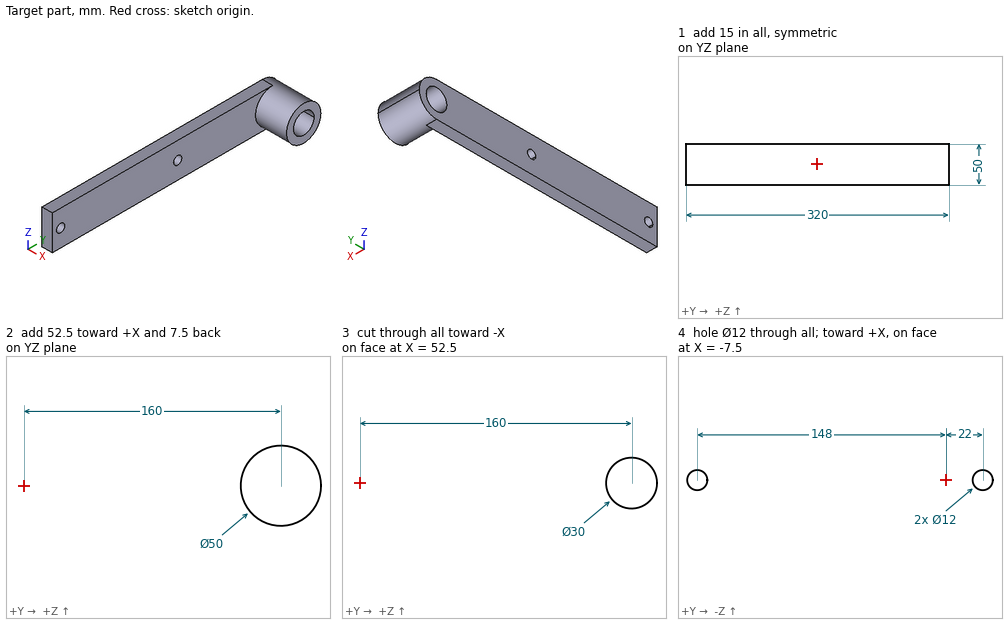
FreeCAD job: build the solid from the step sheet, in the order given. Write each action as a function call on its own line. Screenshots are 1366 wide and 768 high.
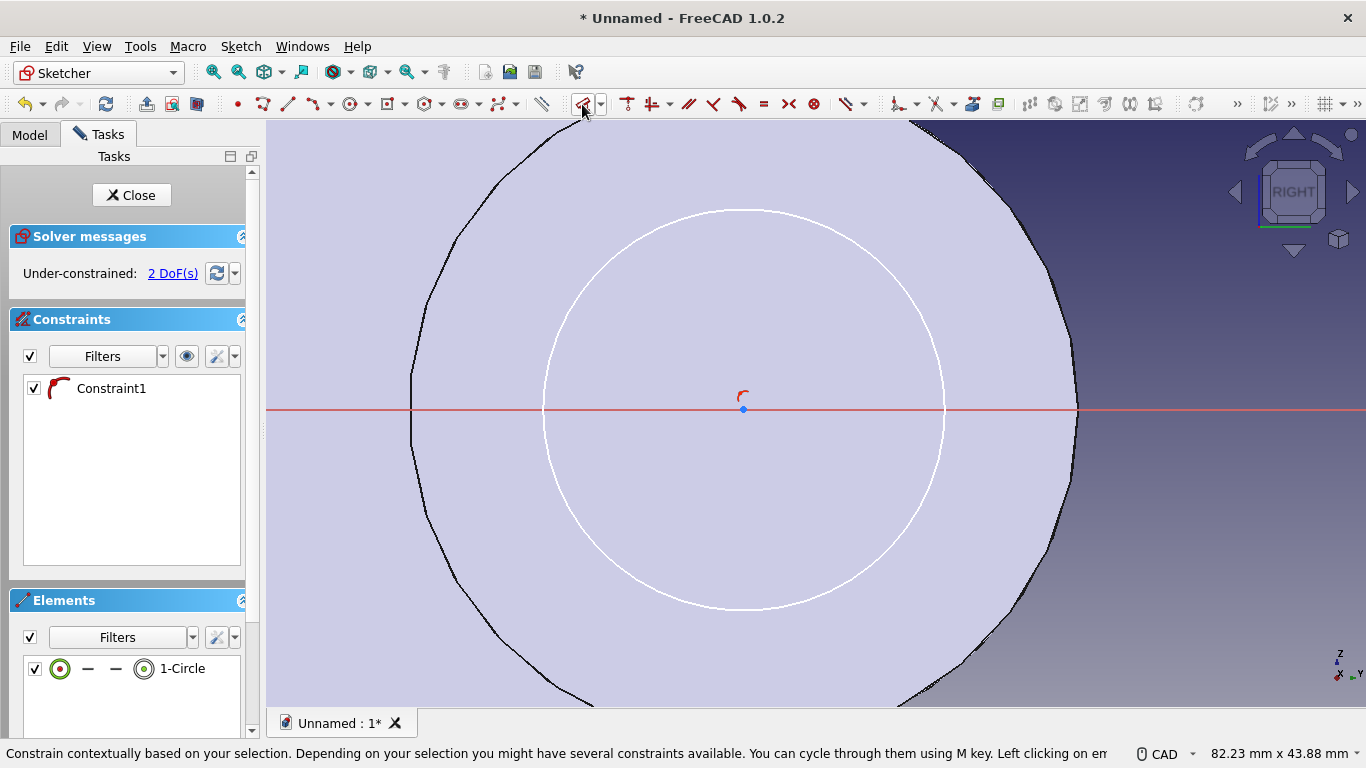
click(886, 268)
click(909, 245)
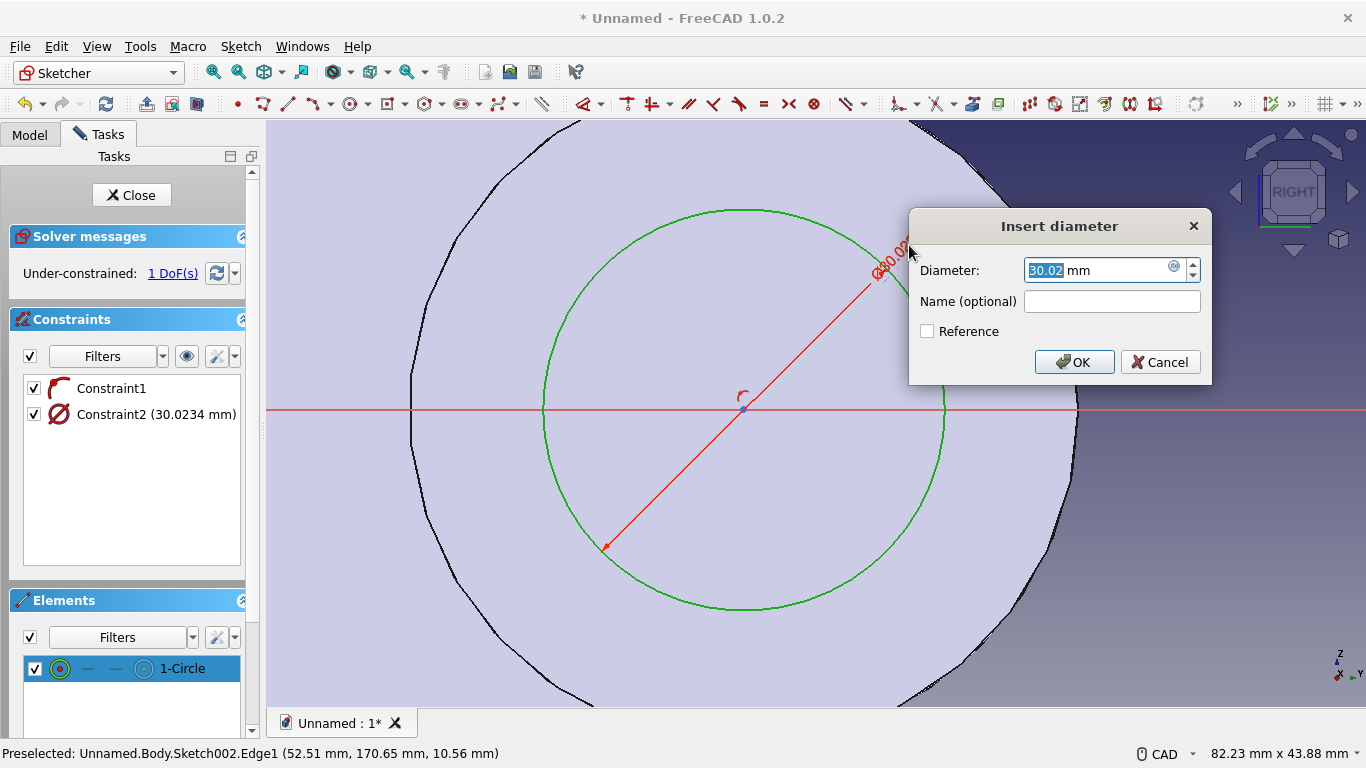
text(30)
key(Return)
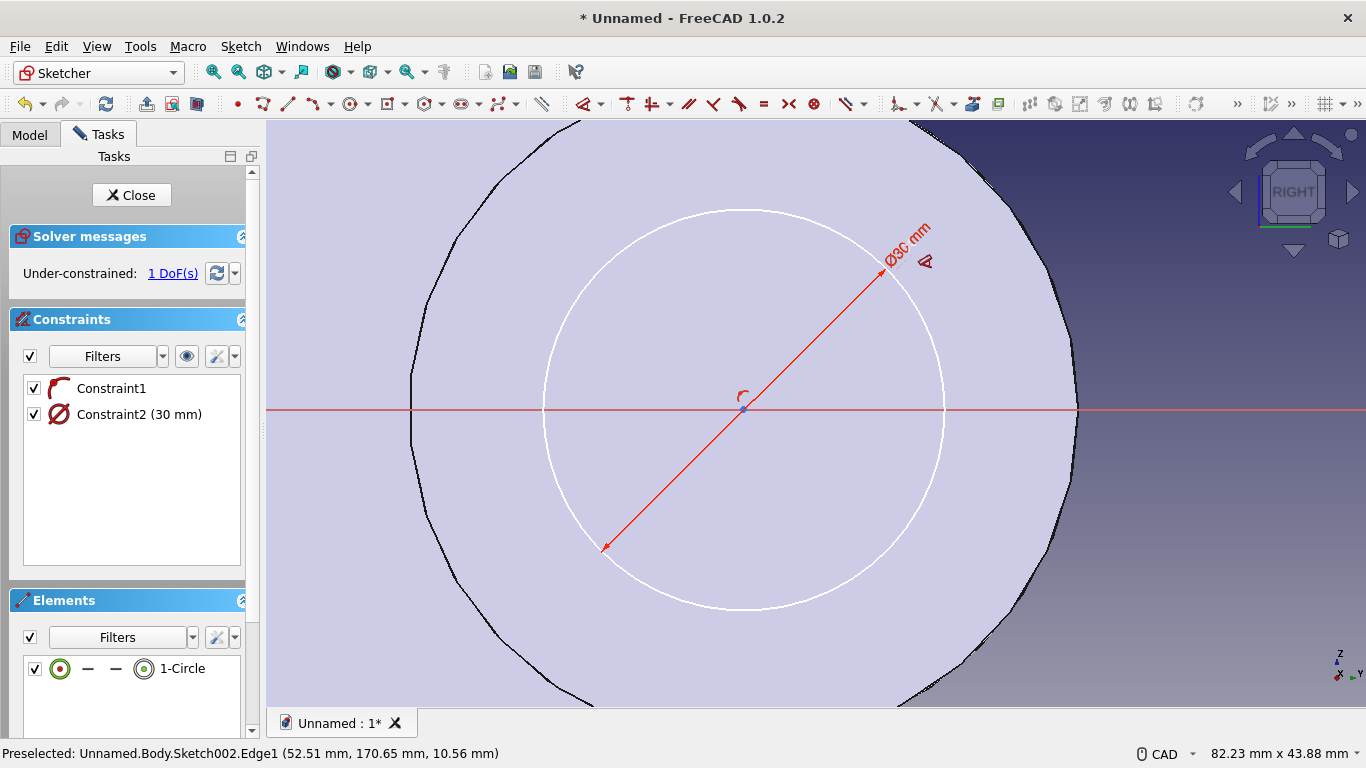
click(744, 410)
click(519, 444)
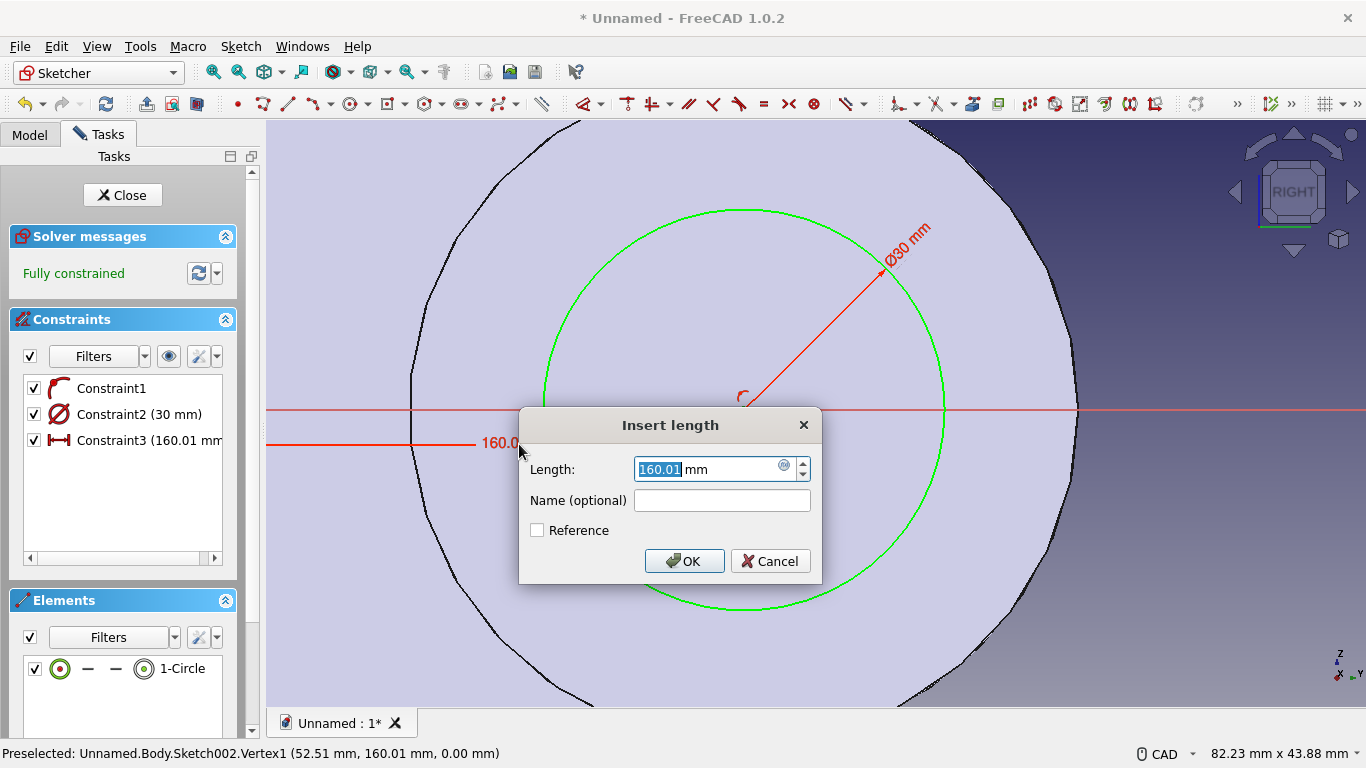
text(160)
key(Return)
key(Escape)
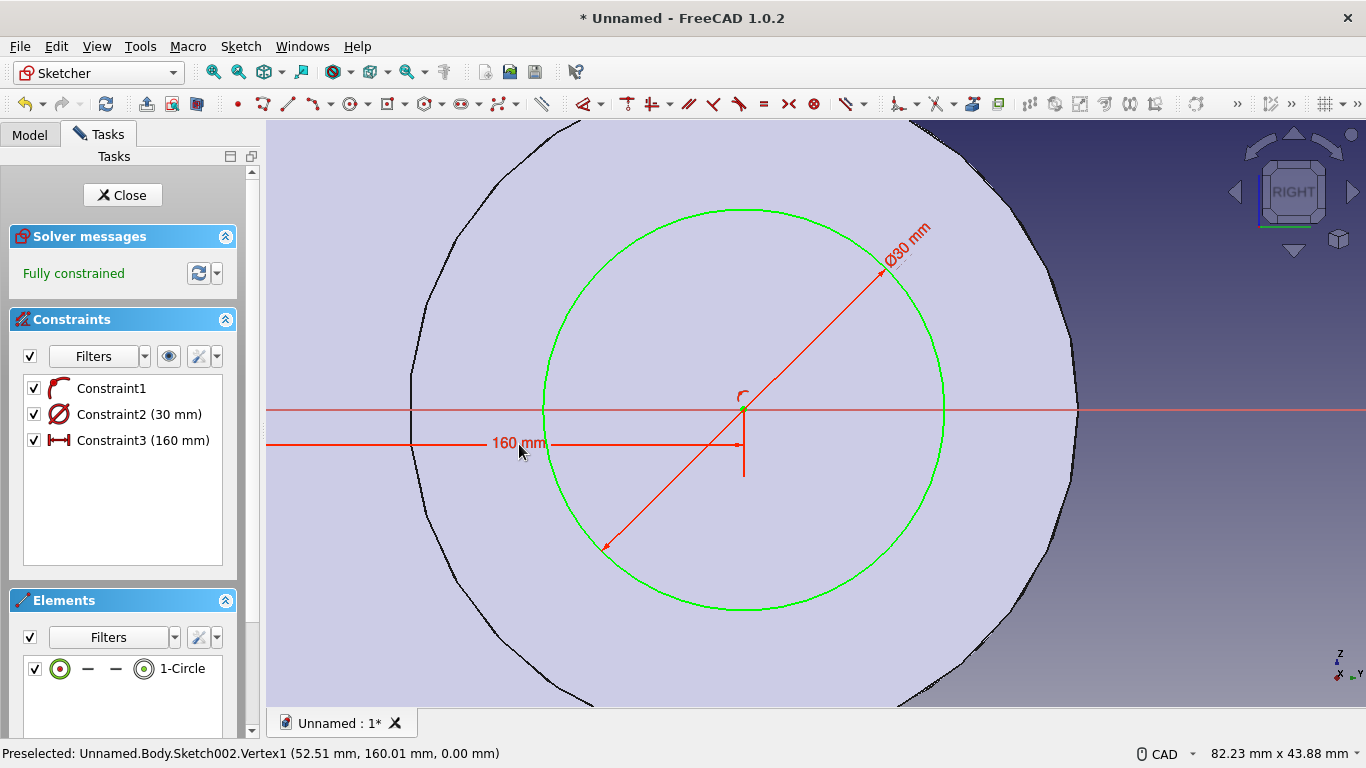
click(123, 195)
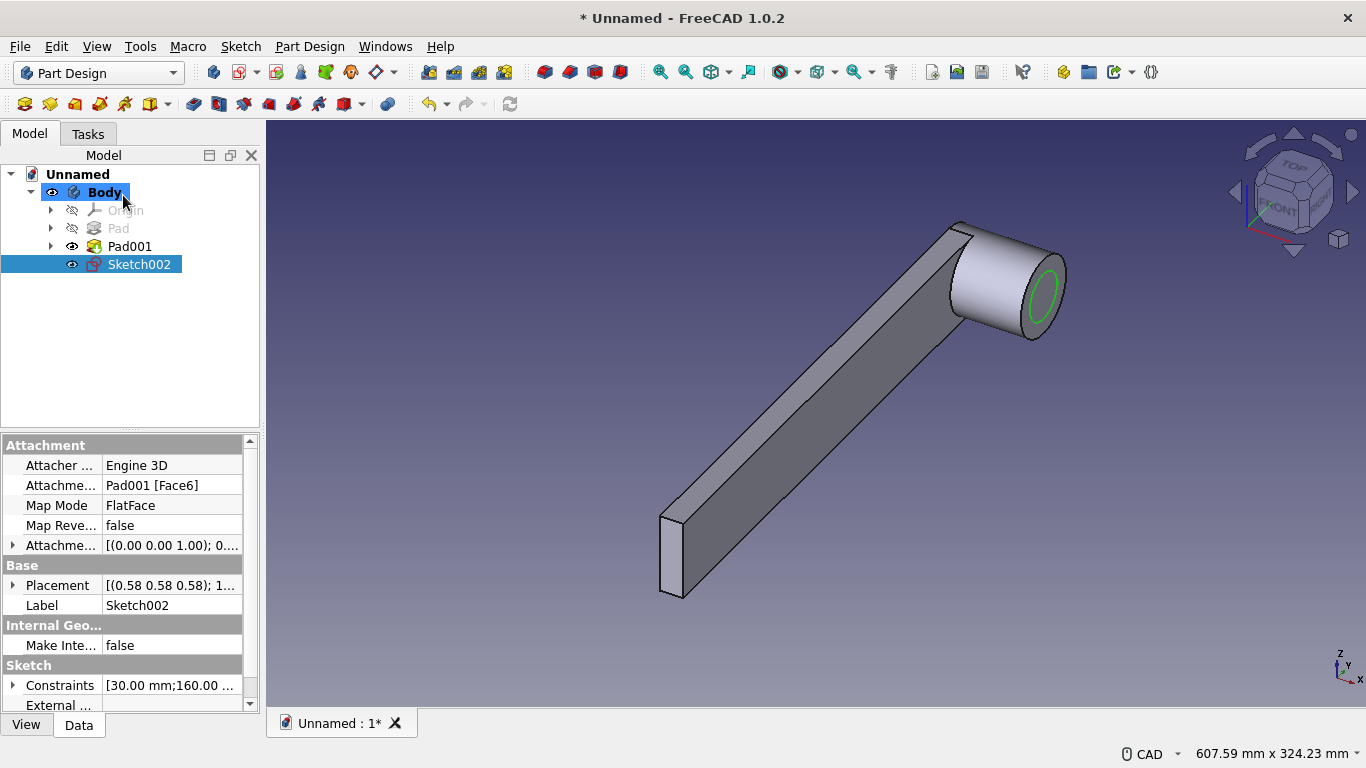
click(194, 104)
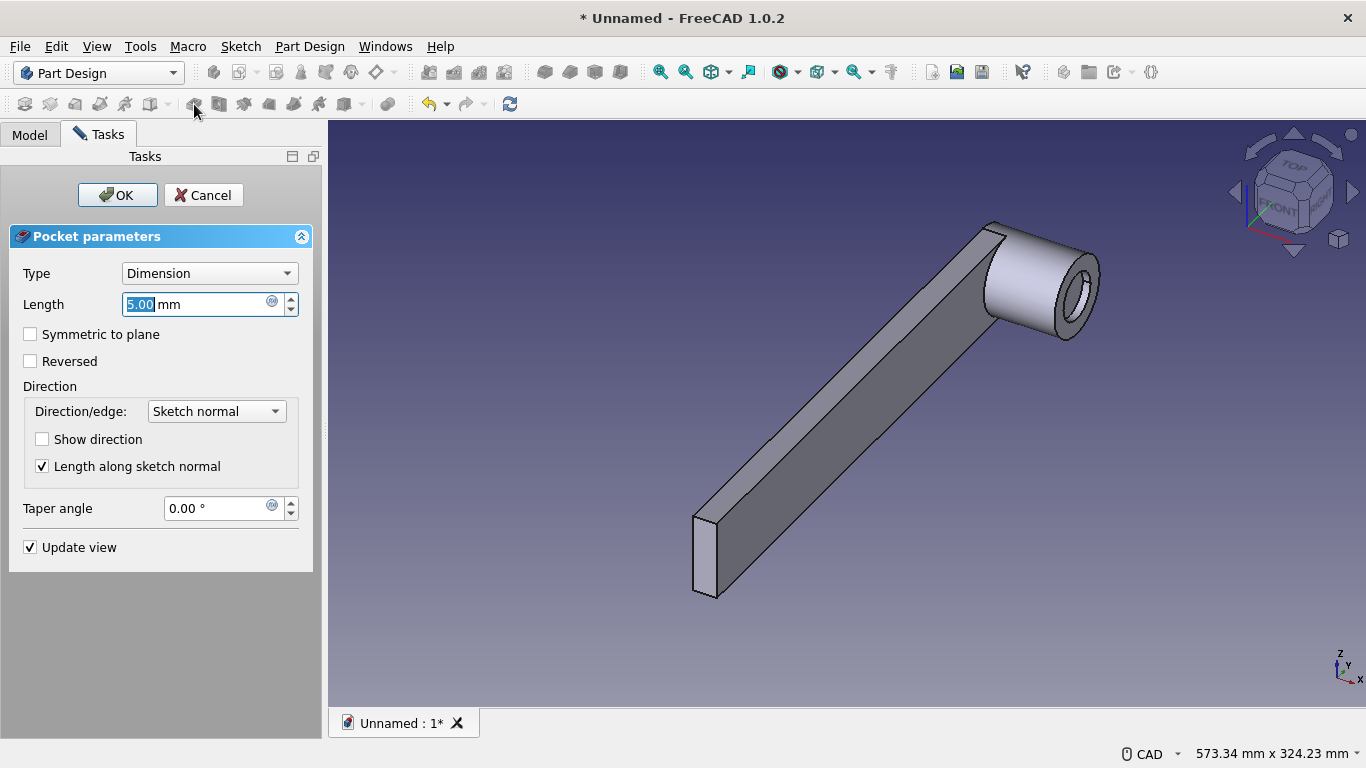
click(210, 274)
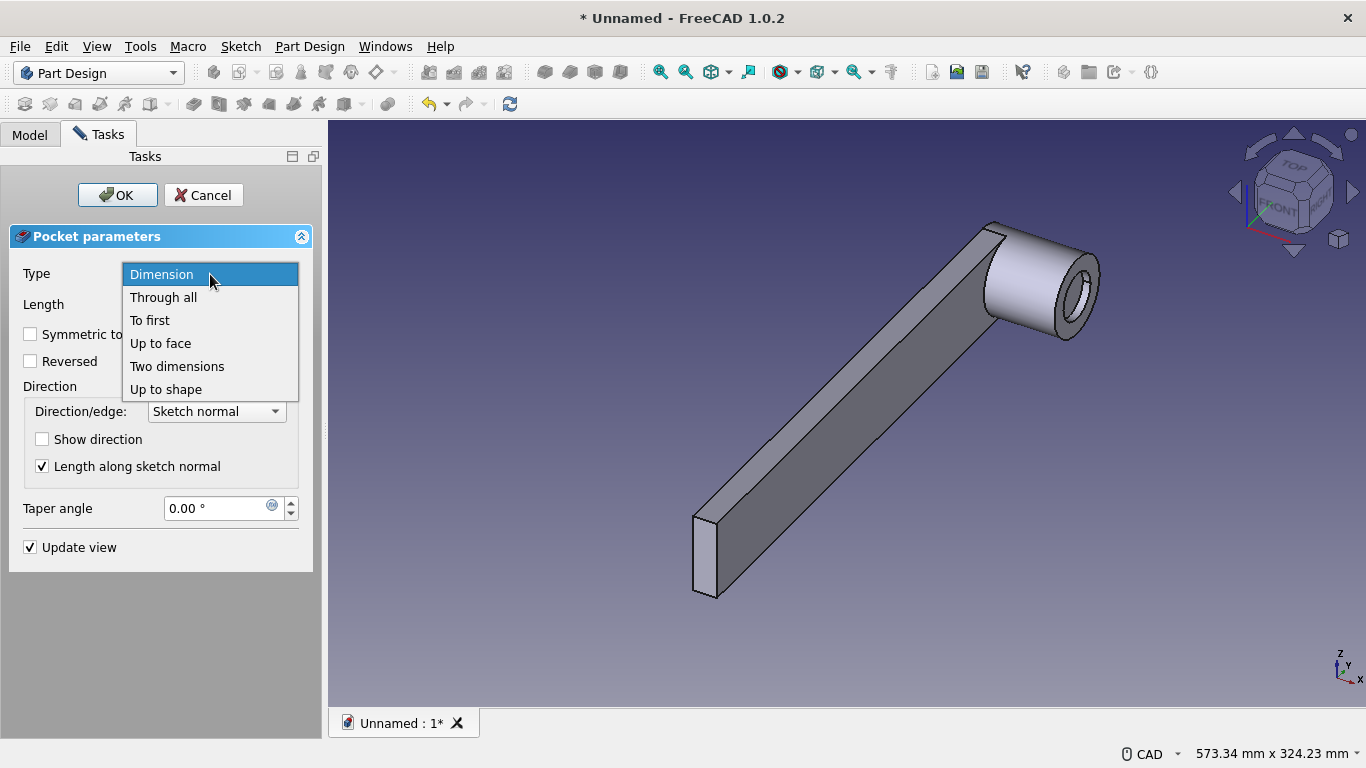
click(208, 298)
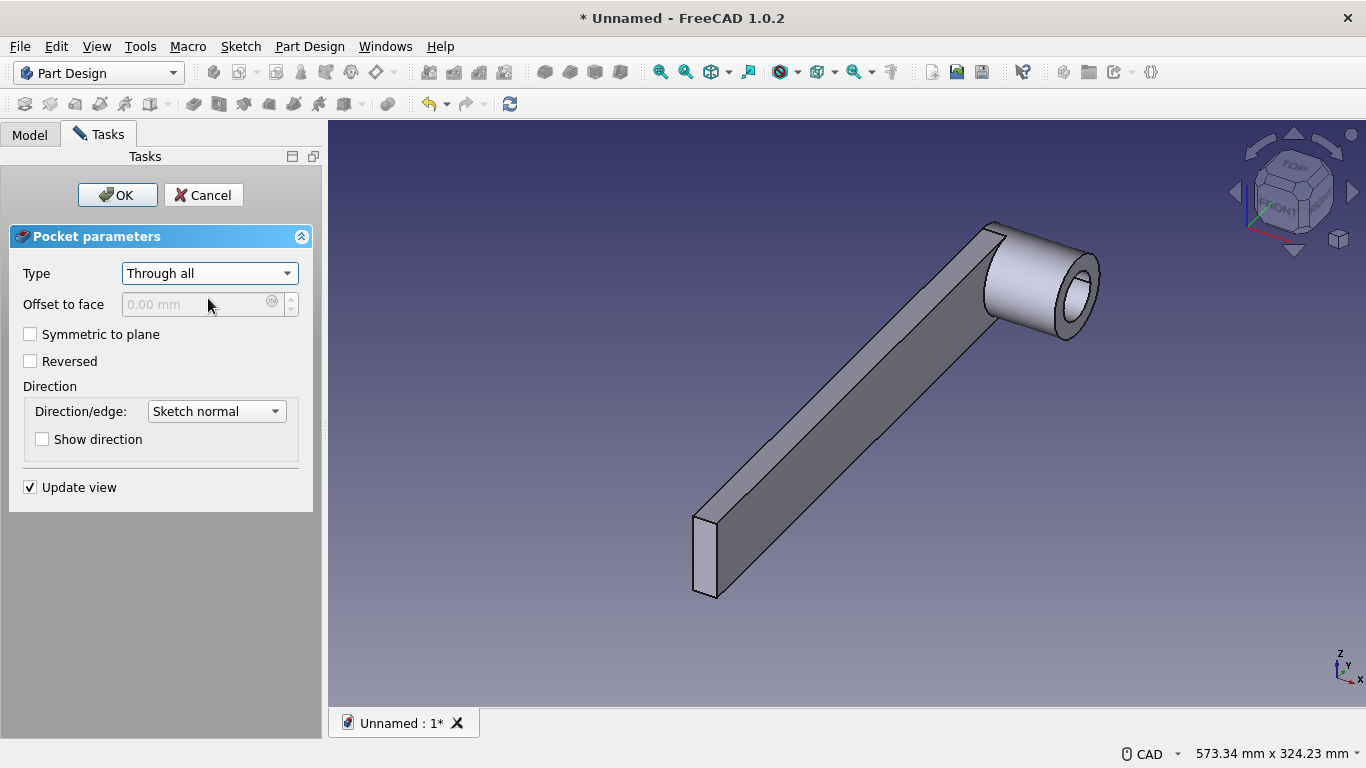
click(118, 195)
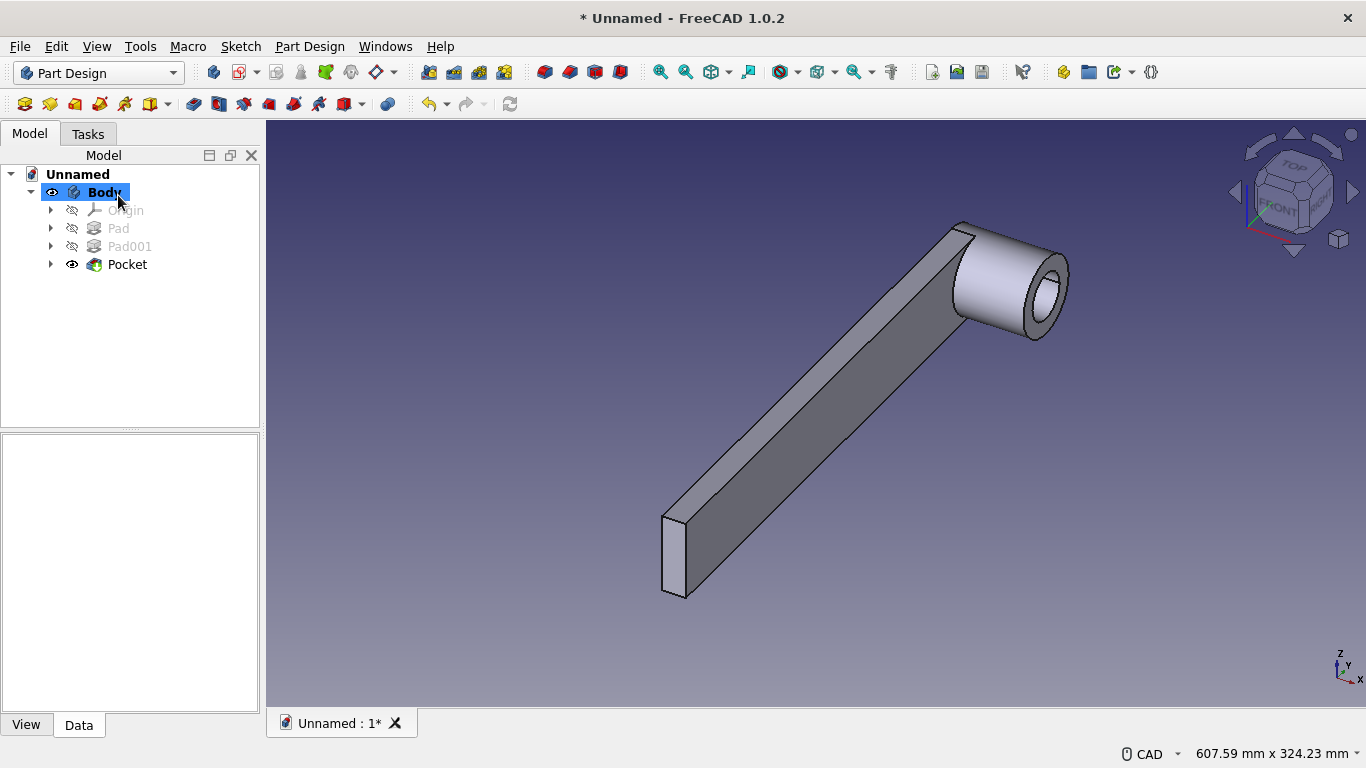
key(6)